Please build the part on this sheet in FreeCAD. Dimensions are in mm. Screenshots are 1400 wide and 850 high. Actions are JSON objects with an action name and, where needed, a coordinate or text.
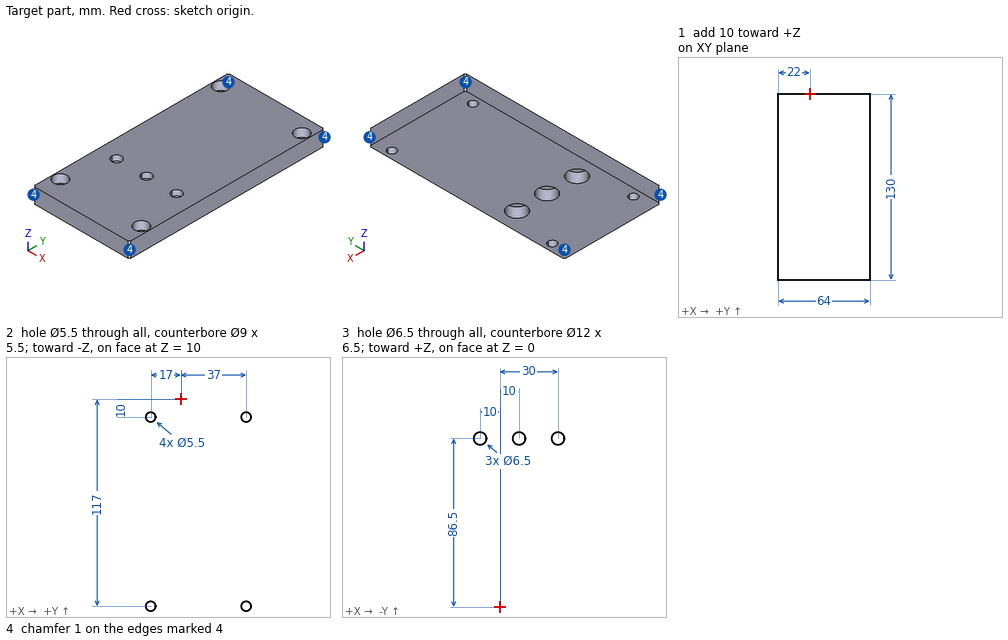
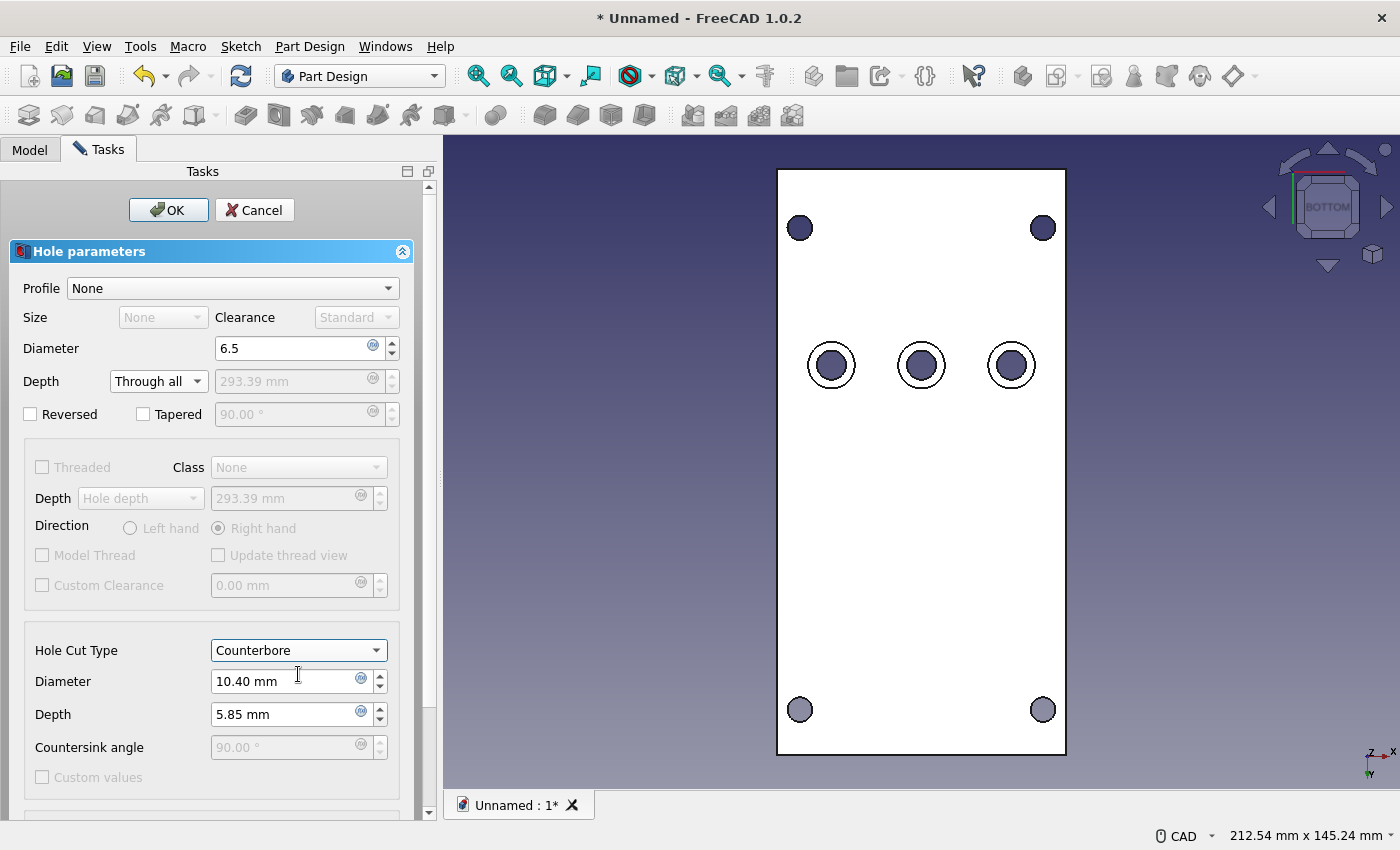
{"action": "triple_click", "coordinate": [292, 682]}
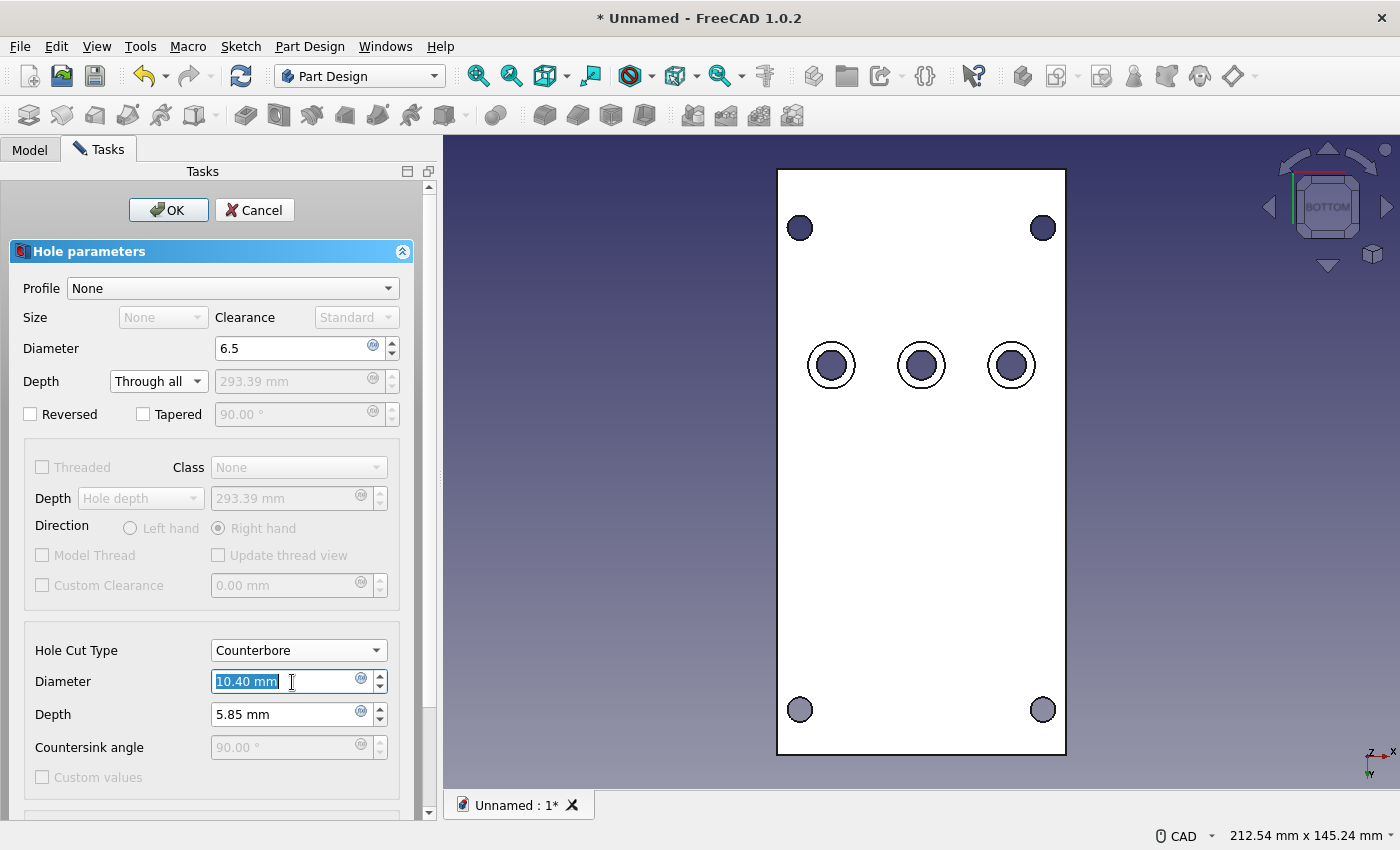
{"action": "type", "text": "12"}
{"action": "key", "text": "Tab"}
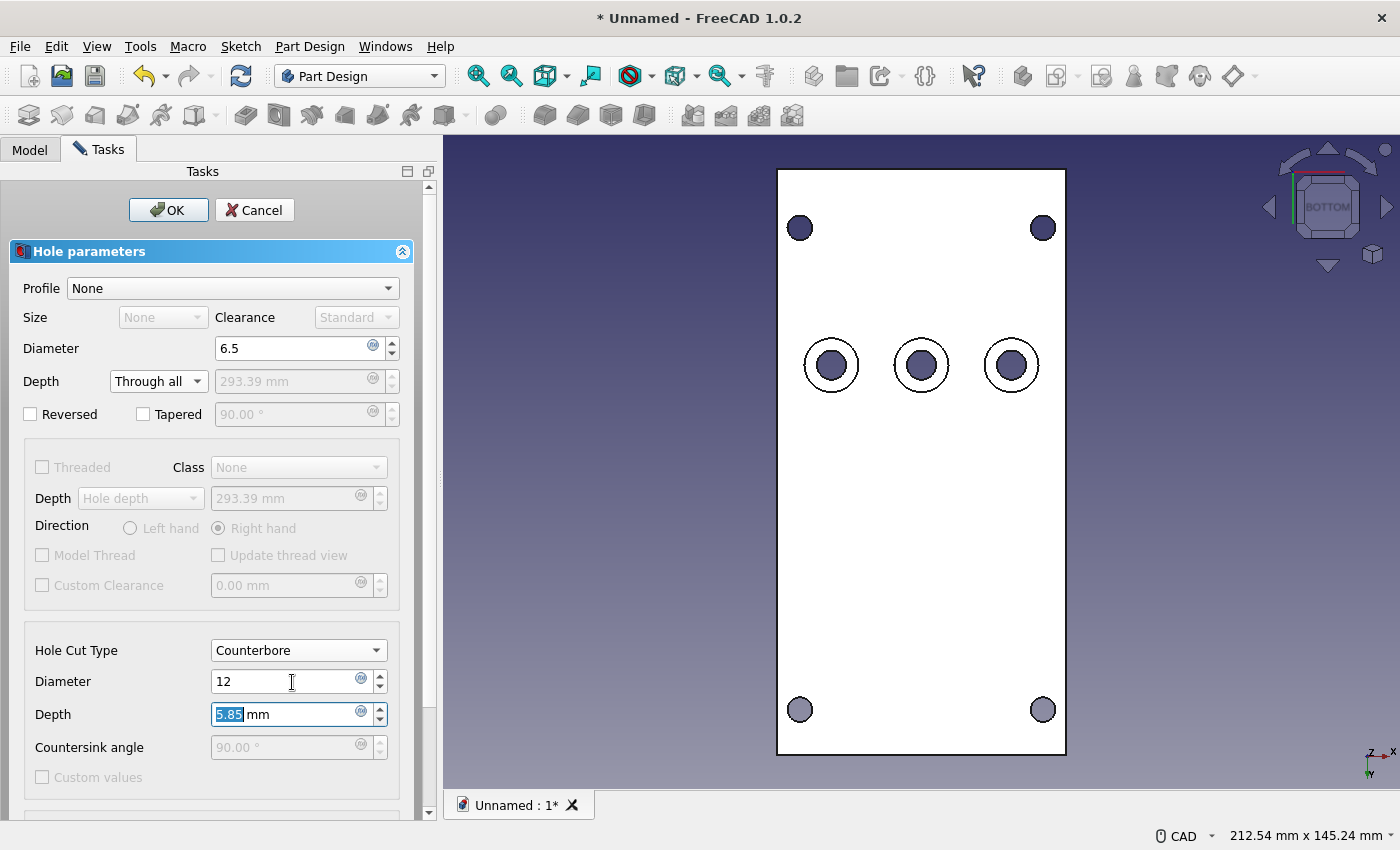
{"action": "type", "text": "6.5"}
{"action": "key", "text": "Tab"}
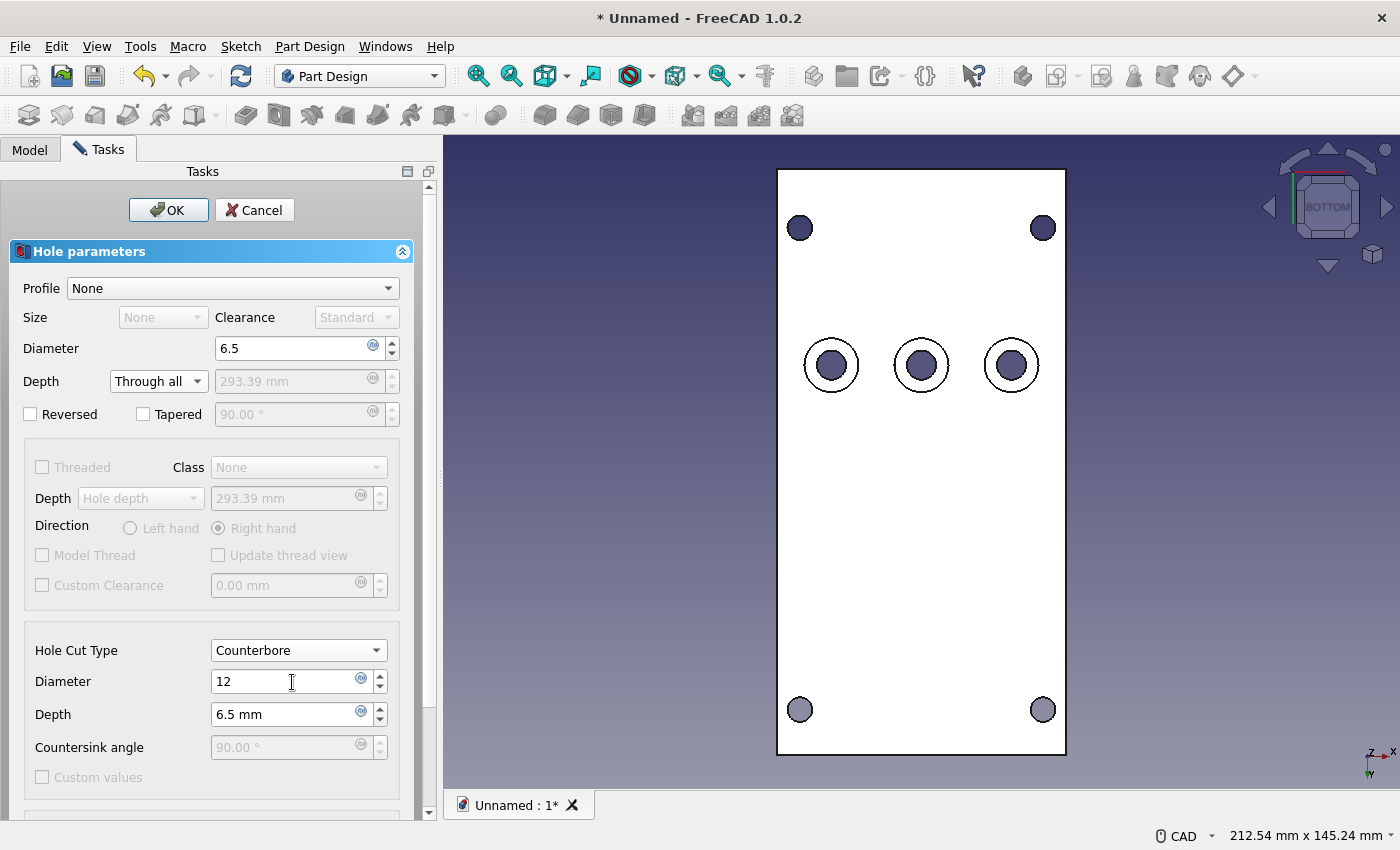
{"action": "left_click", "coordinate": [169, 210]}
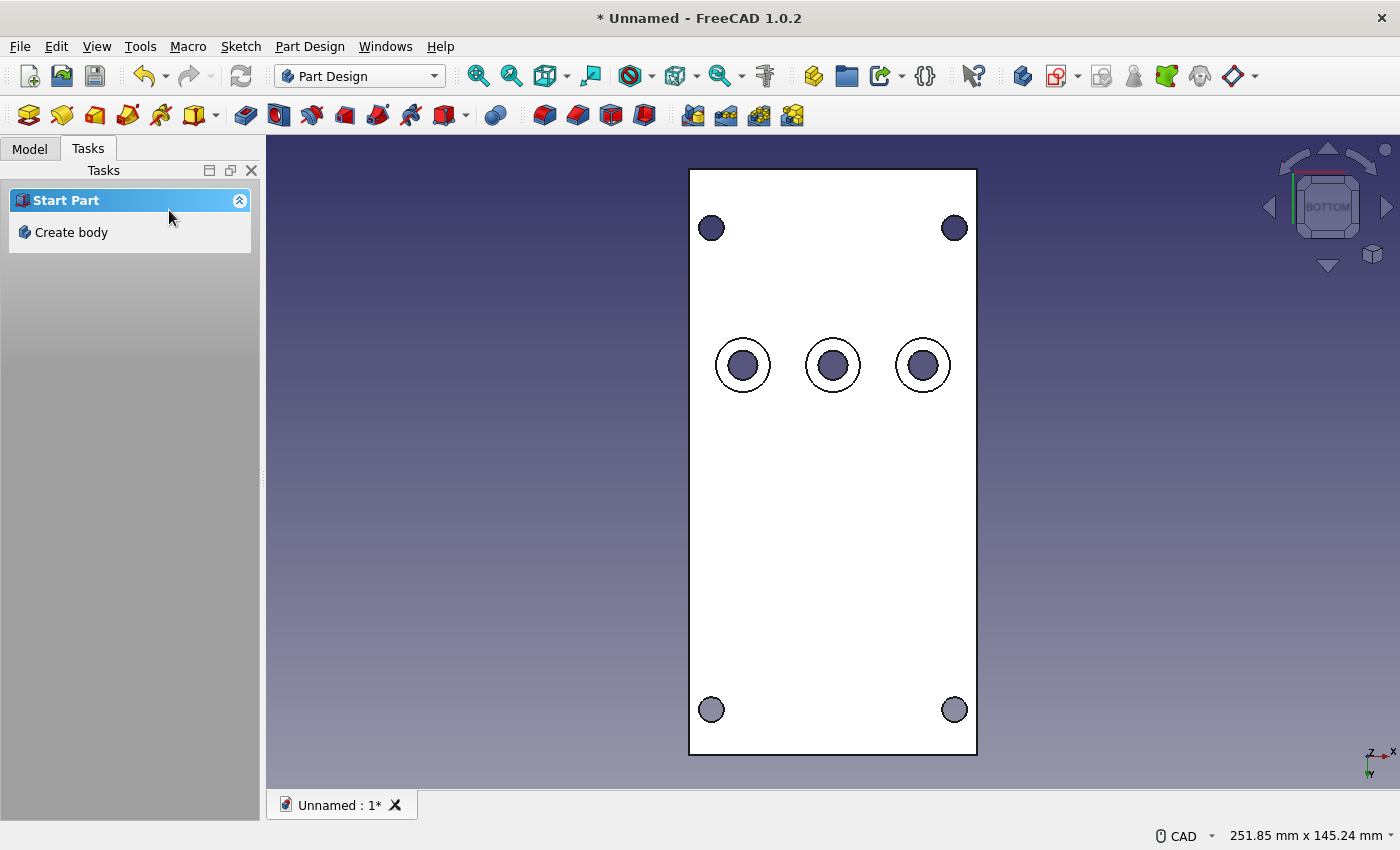
{"action": "key", "text": "0"}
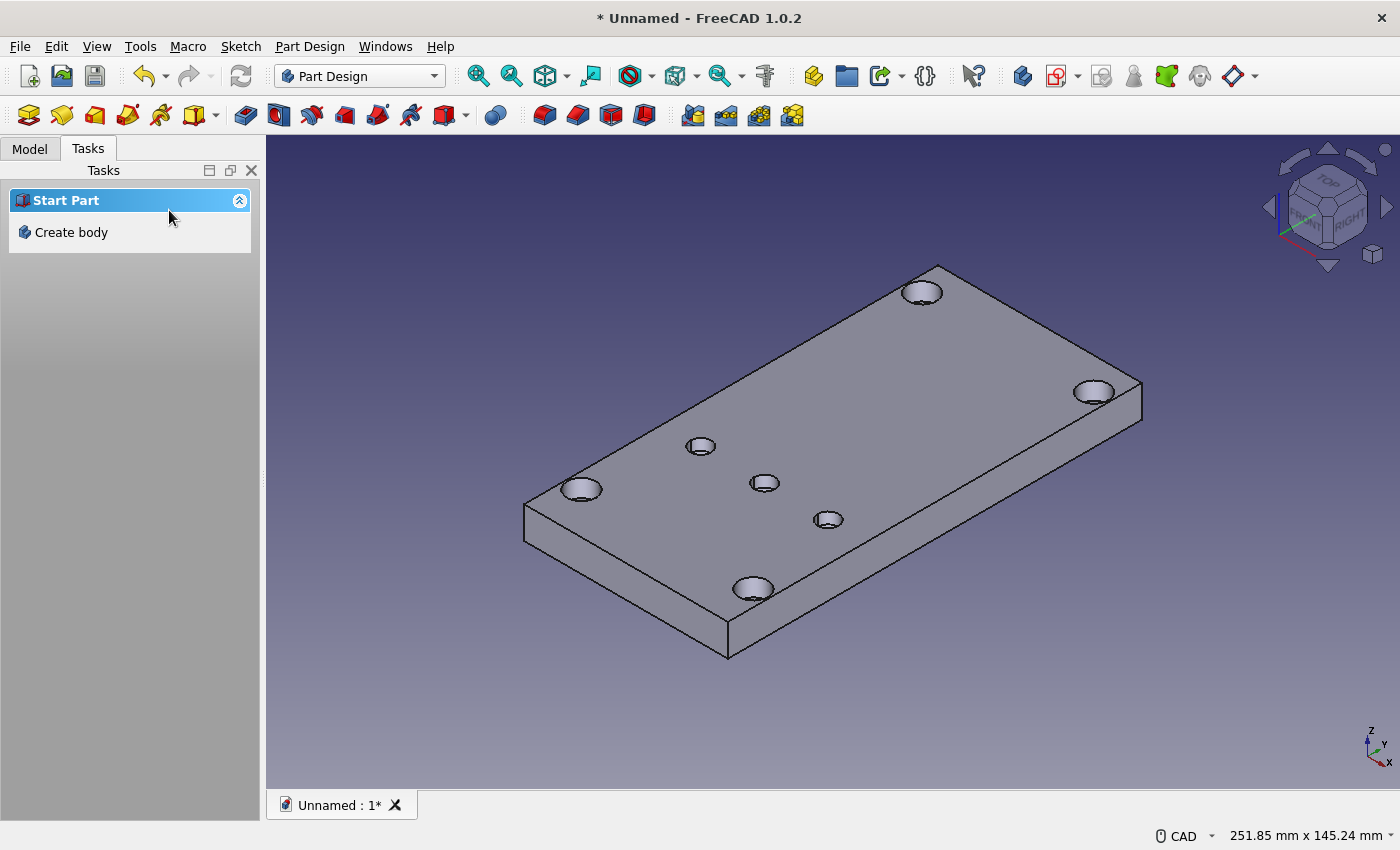
{"action": "left_click", "coordinate": [728, 639]}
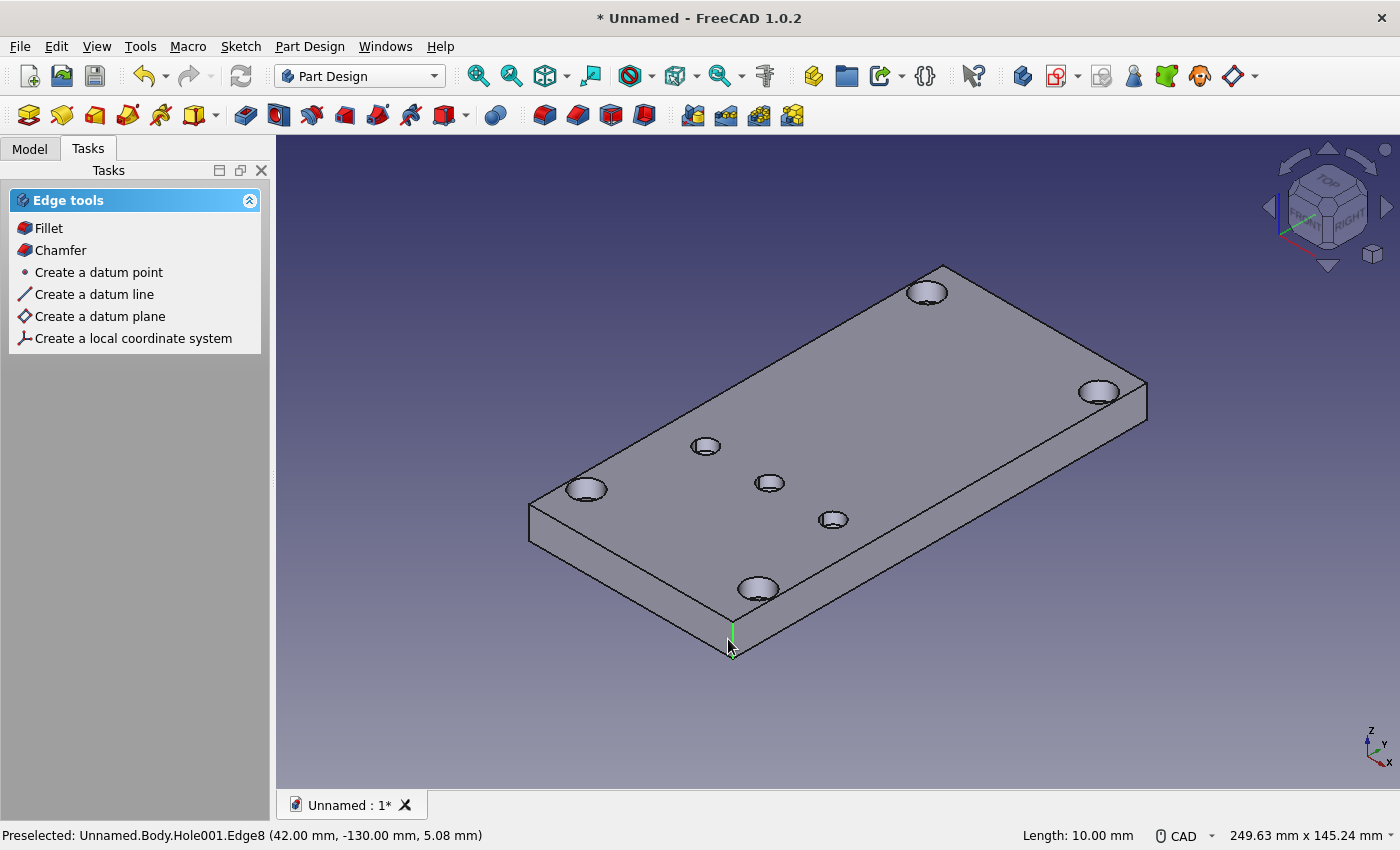
{"action": "key", "text": "2"}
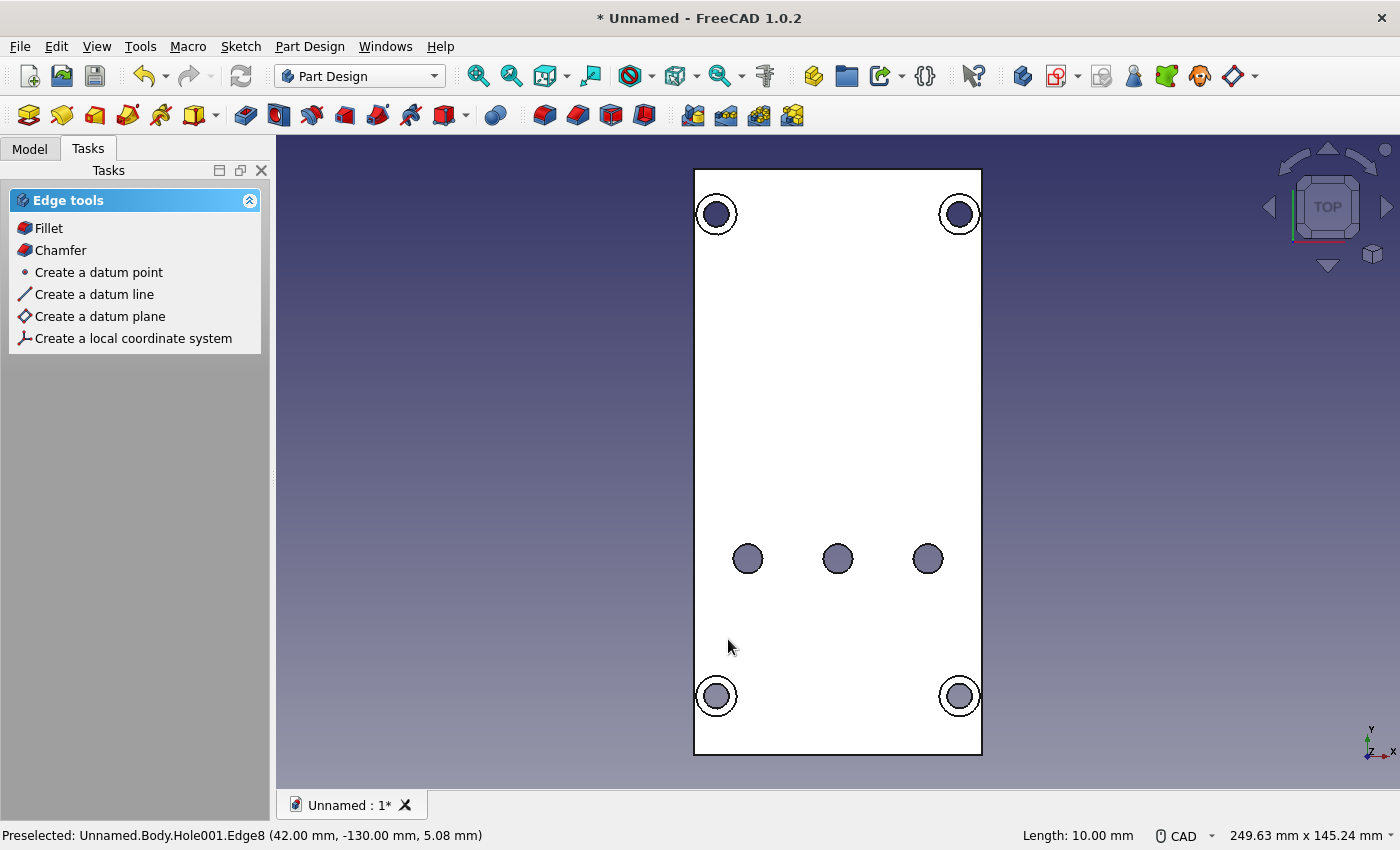
{"action": "key", "text": "1"}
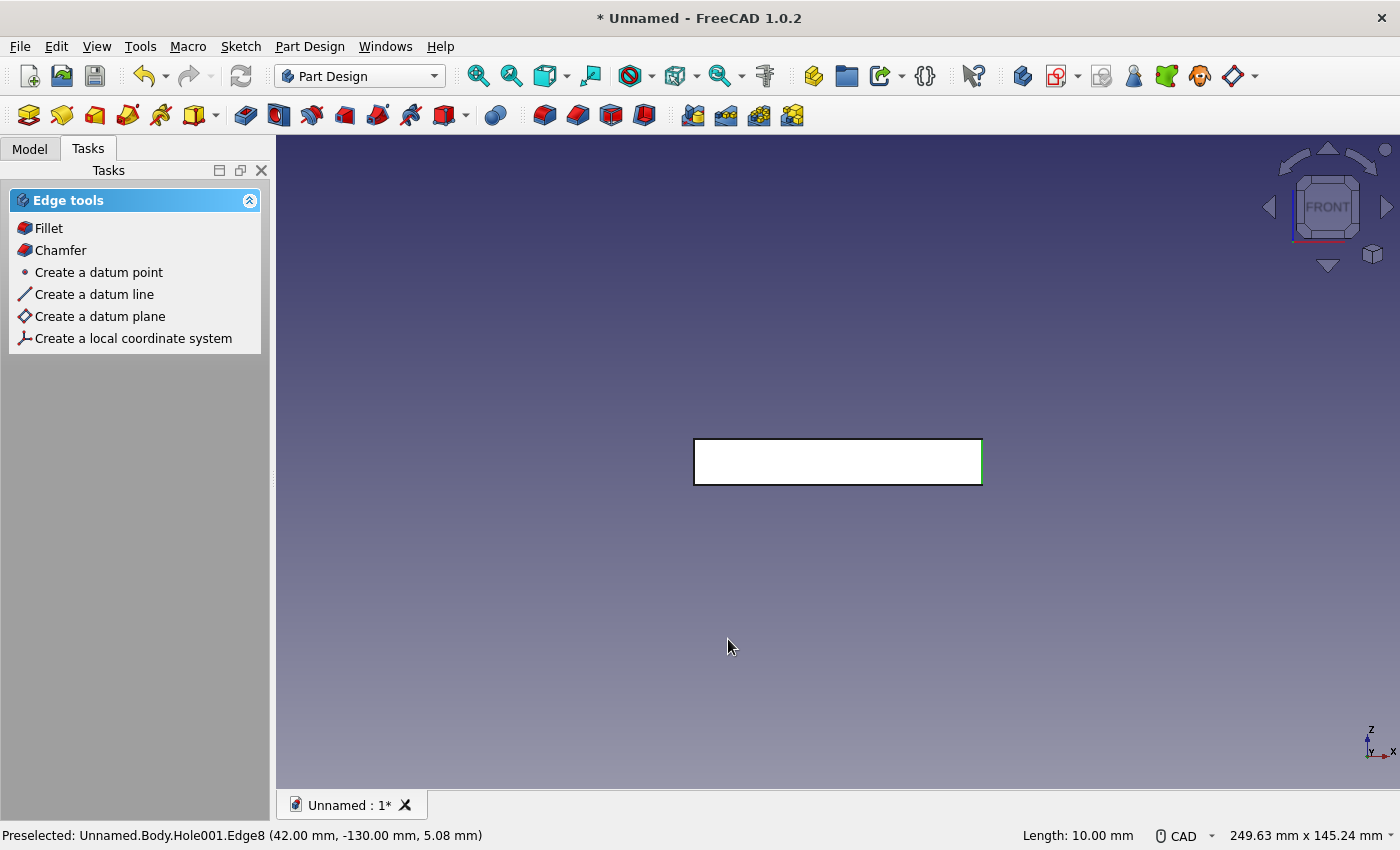
{"action": "key", "text": "v f"}